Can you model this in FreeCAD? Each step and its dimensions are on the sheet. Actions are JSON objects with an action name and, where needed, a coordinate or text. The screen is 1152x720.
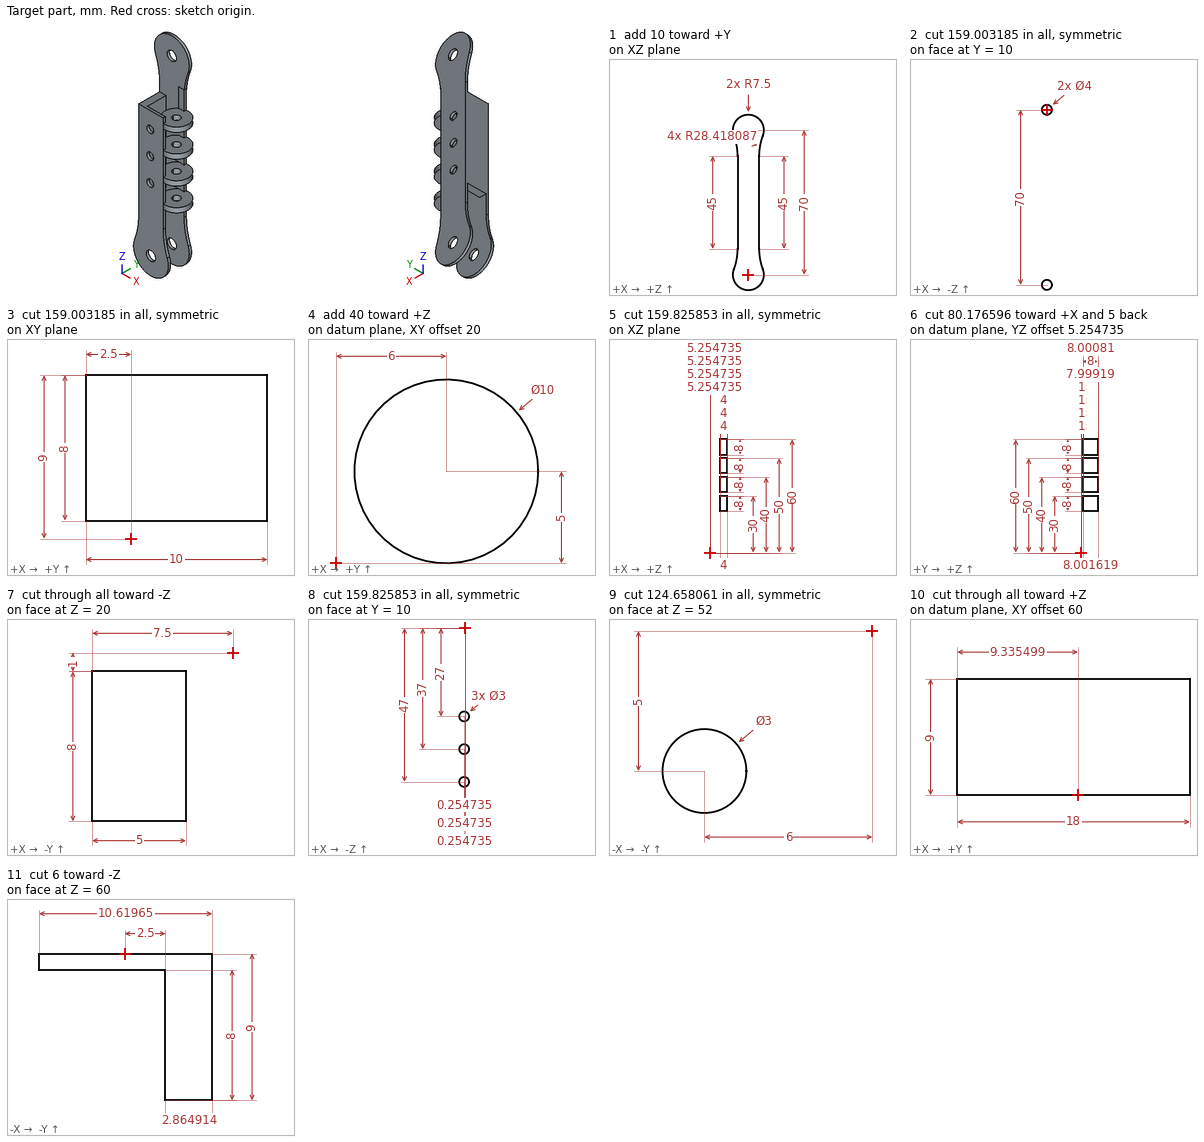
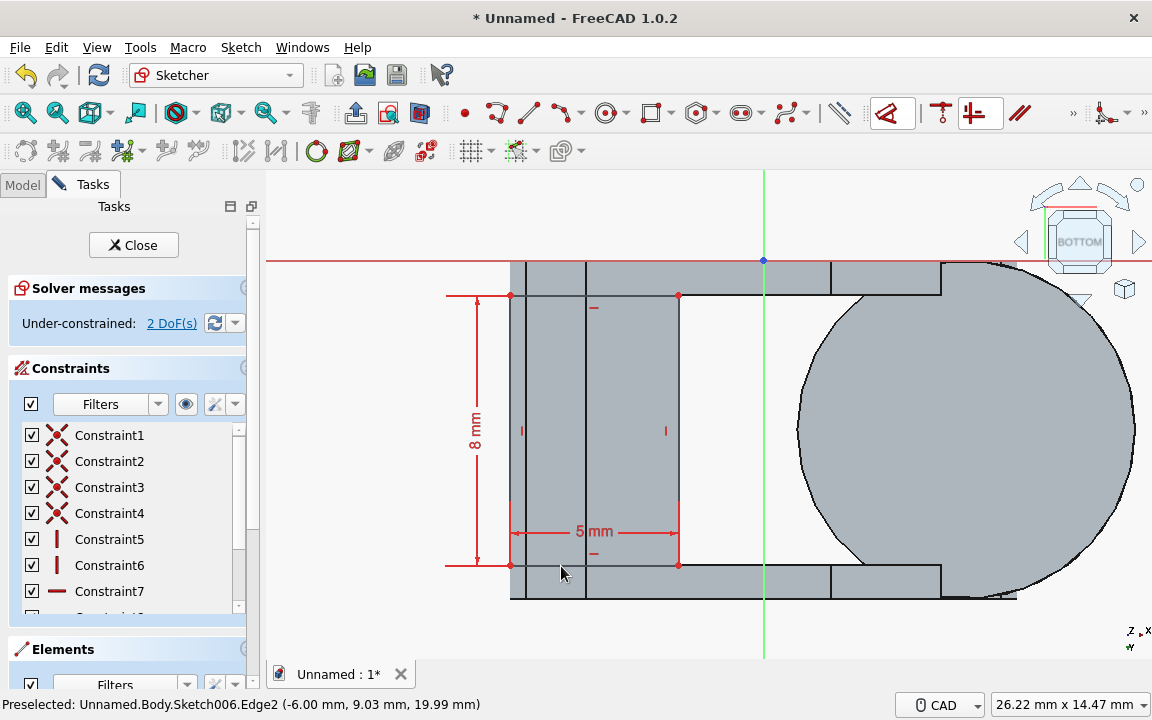
{"action": "left_click", "coordinate": [510, 296]}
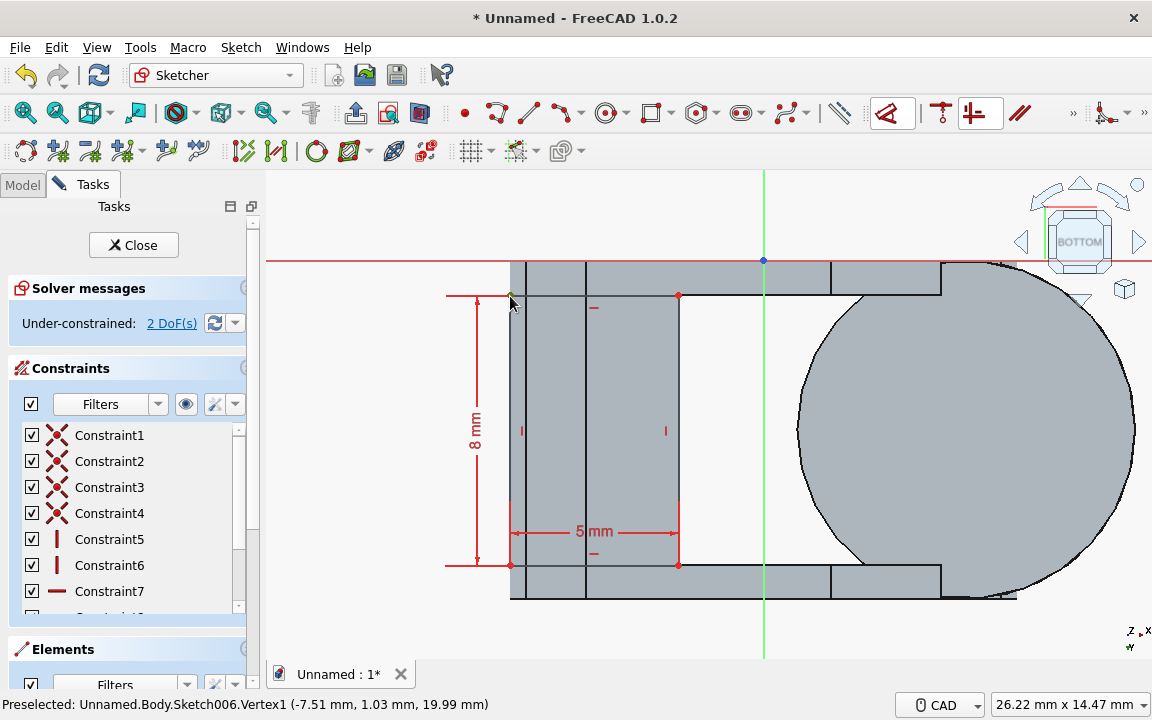
{"action": "left_click", "coordinate": [910, 114]}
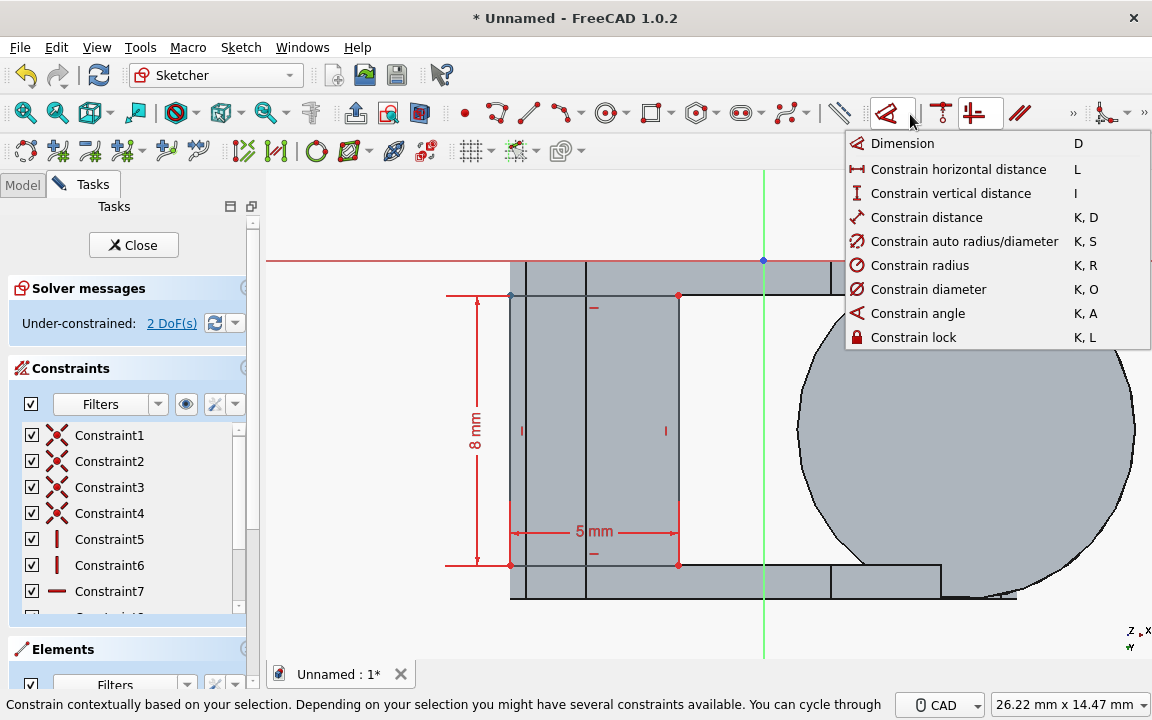
{"action": "left_click", "coordinate": [998, 193]}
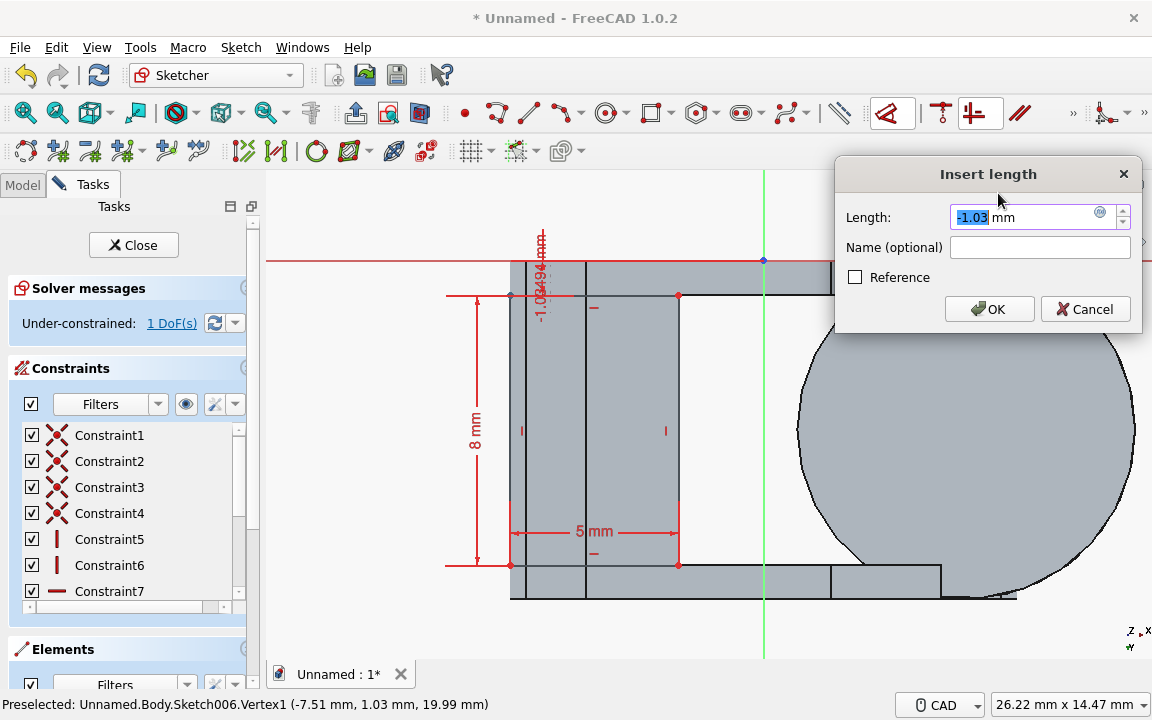
{"action": "type", "text": "-1"}
{"action": "key", "text": "Return"}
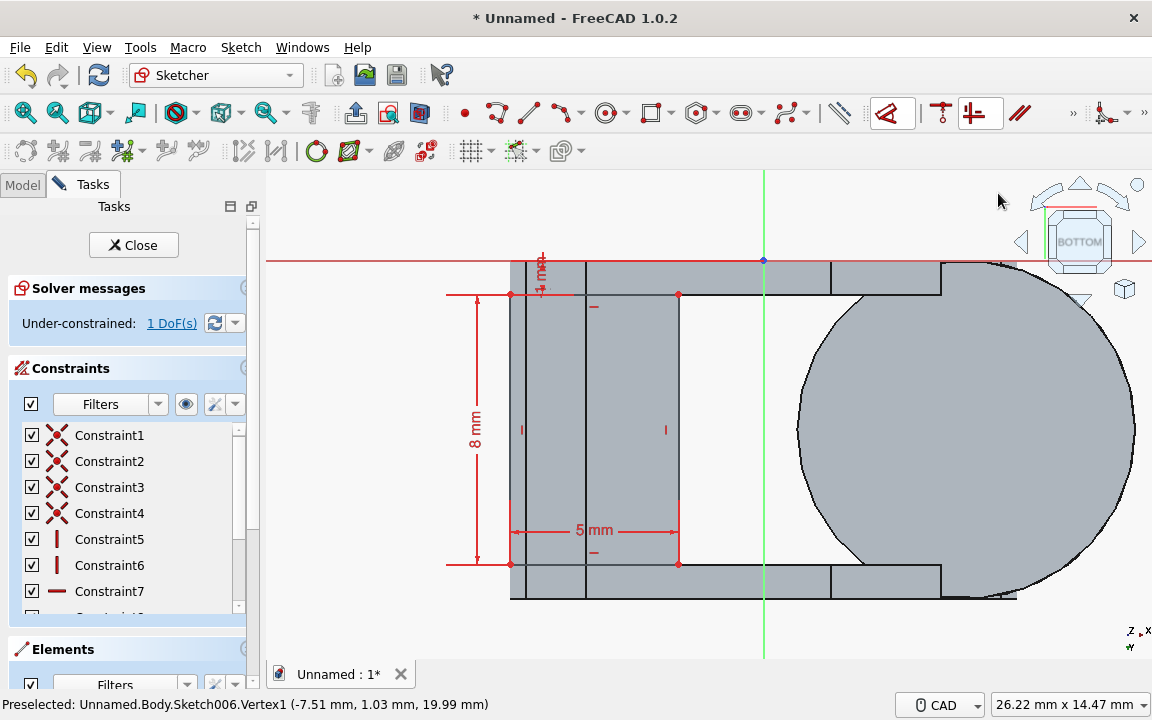
{"action": "left_click", "coordinate": [510, 295]}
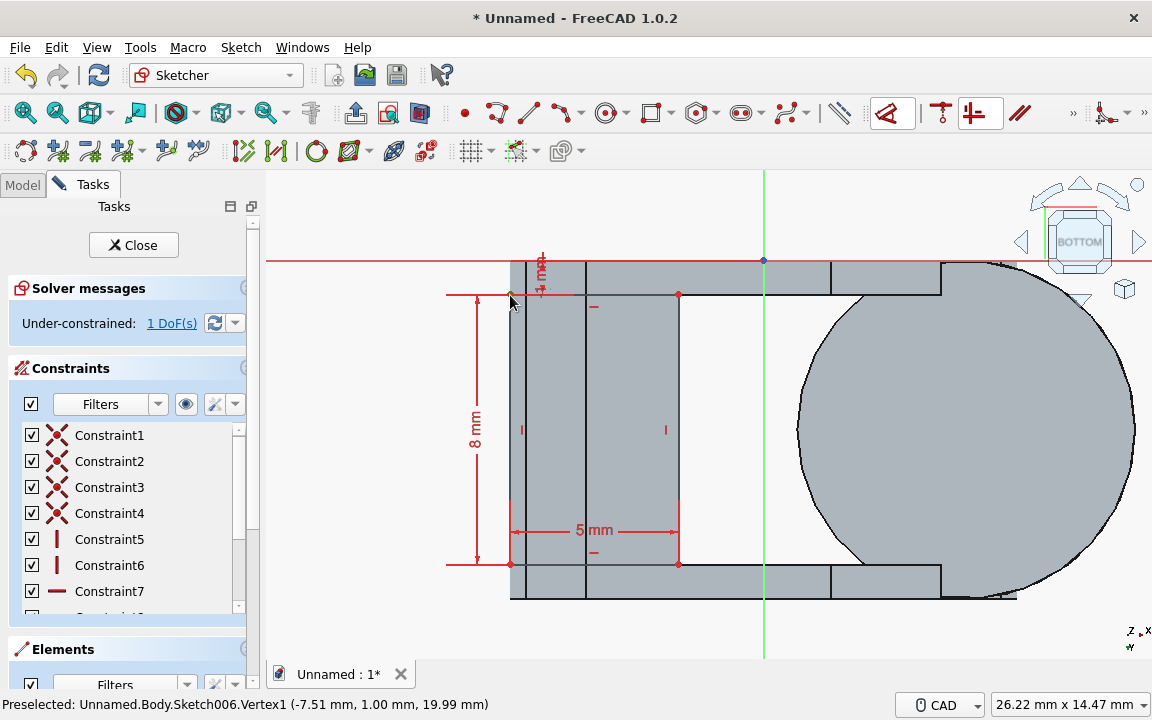
{"action": "key", "text": "l"}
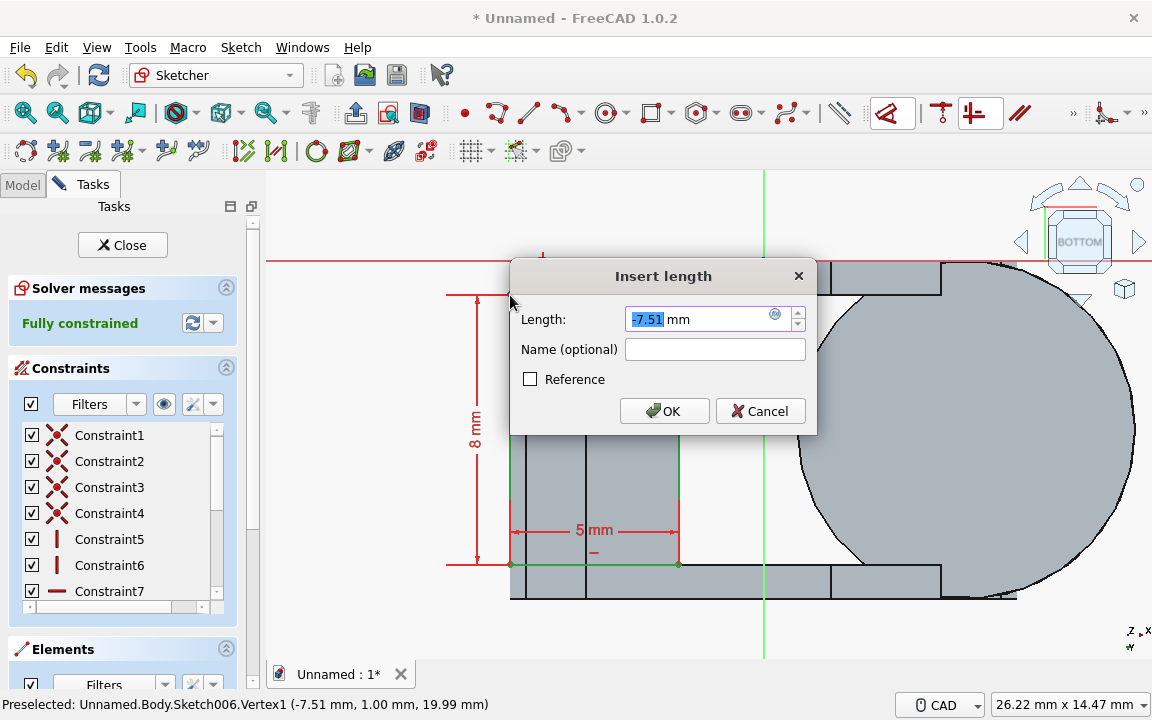
{"action": "type", "text": "-7.5"}
{"action": "key", "text": "Return"}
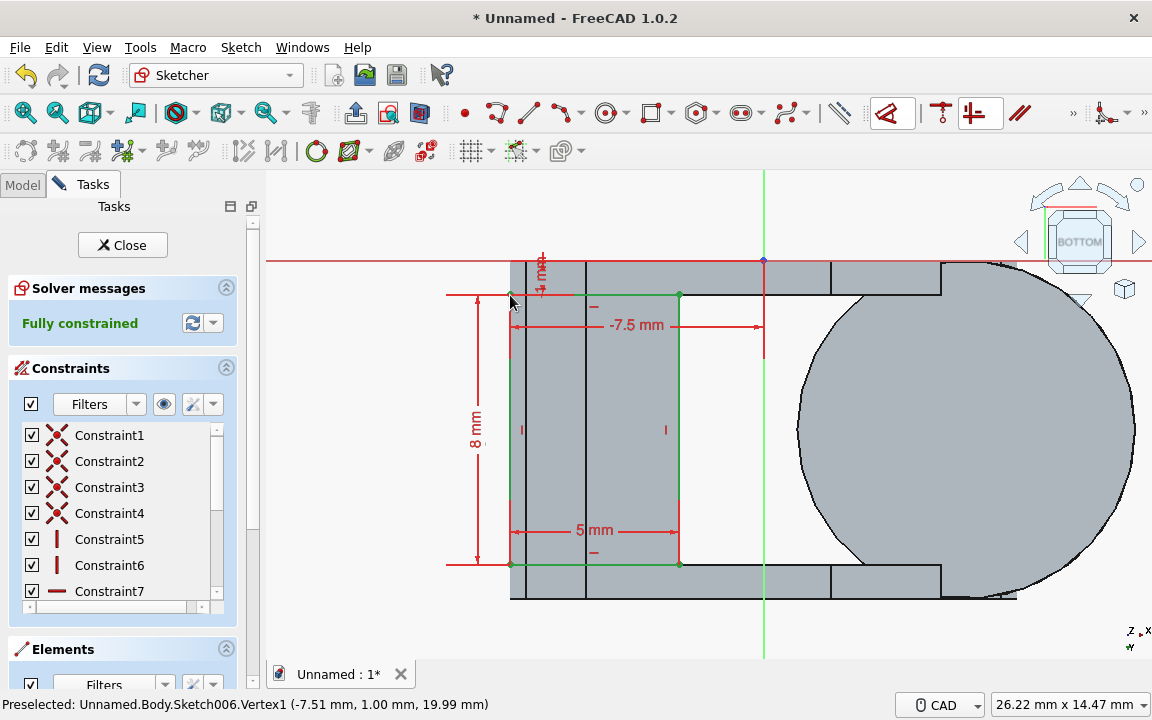
{"action": "left_click", "coordinate": [123, 245]}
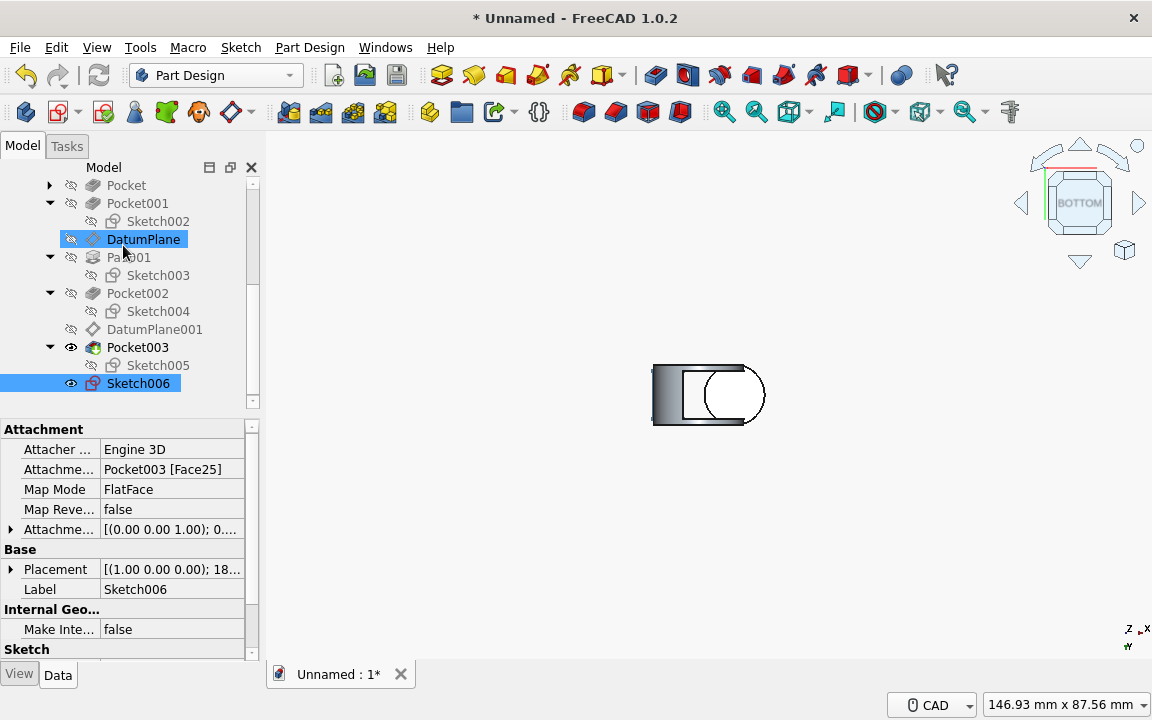
{"action": "left_click", "coordinate": [656, 76]}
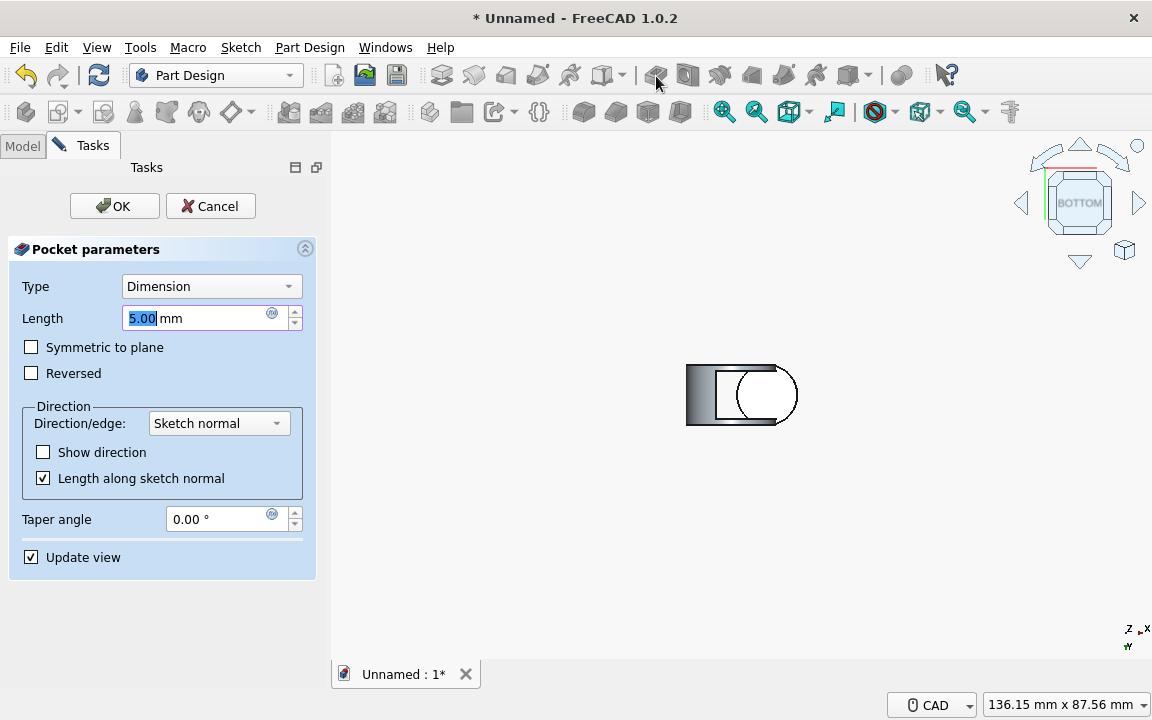
{"action": "left_click", "coordinate": [212, 286]}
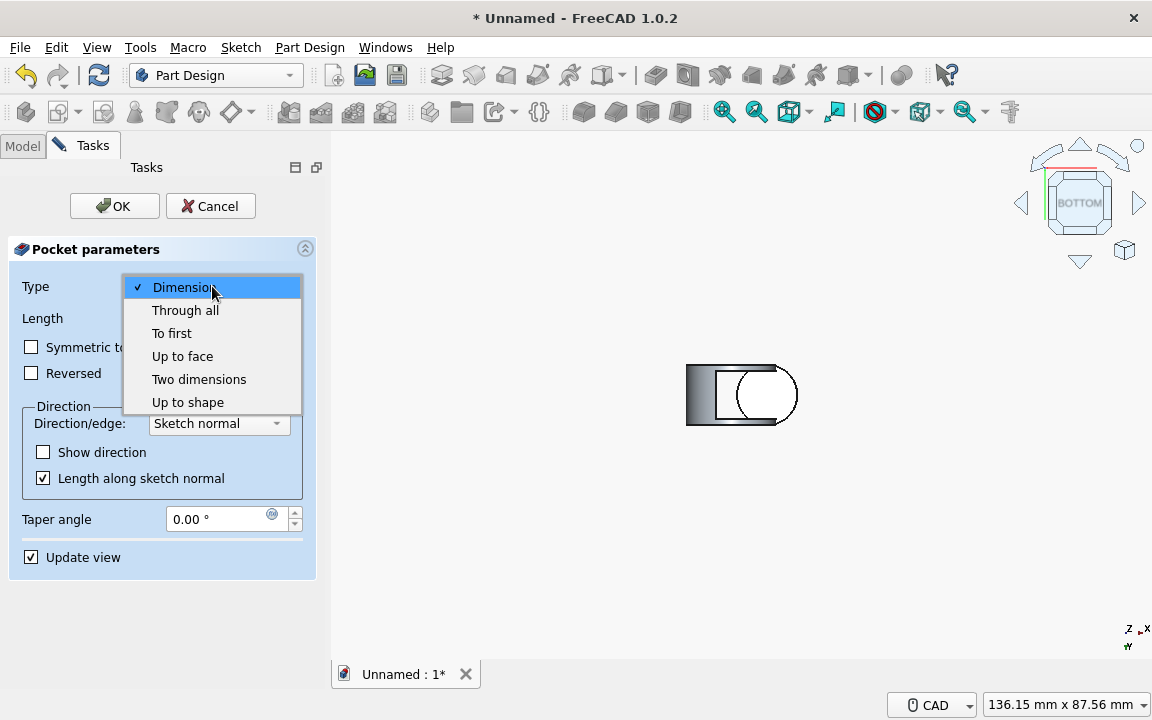
{"action": "left_click", "coordinate": [212, 310]}